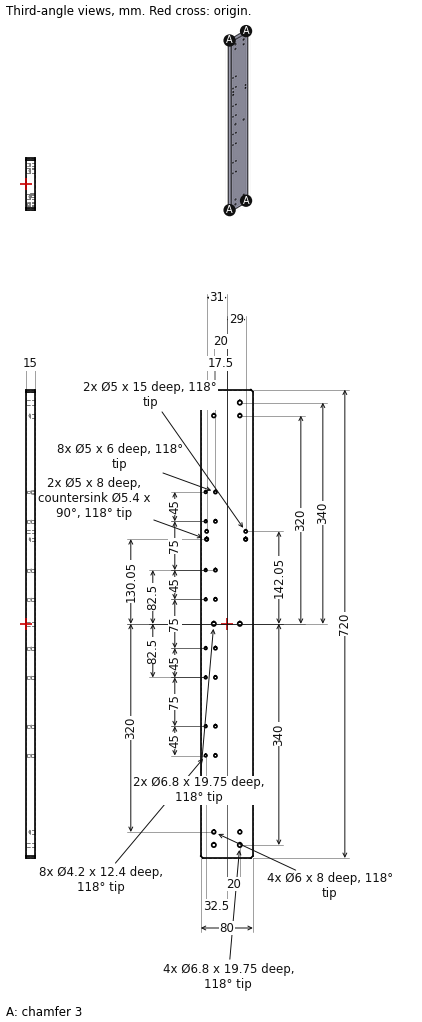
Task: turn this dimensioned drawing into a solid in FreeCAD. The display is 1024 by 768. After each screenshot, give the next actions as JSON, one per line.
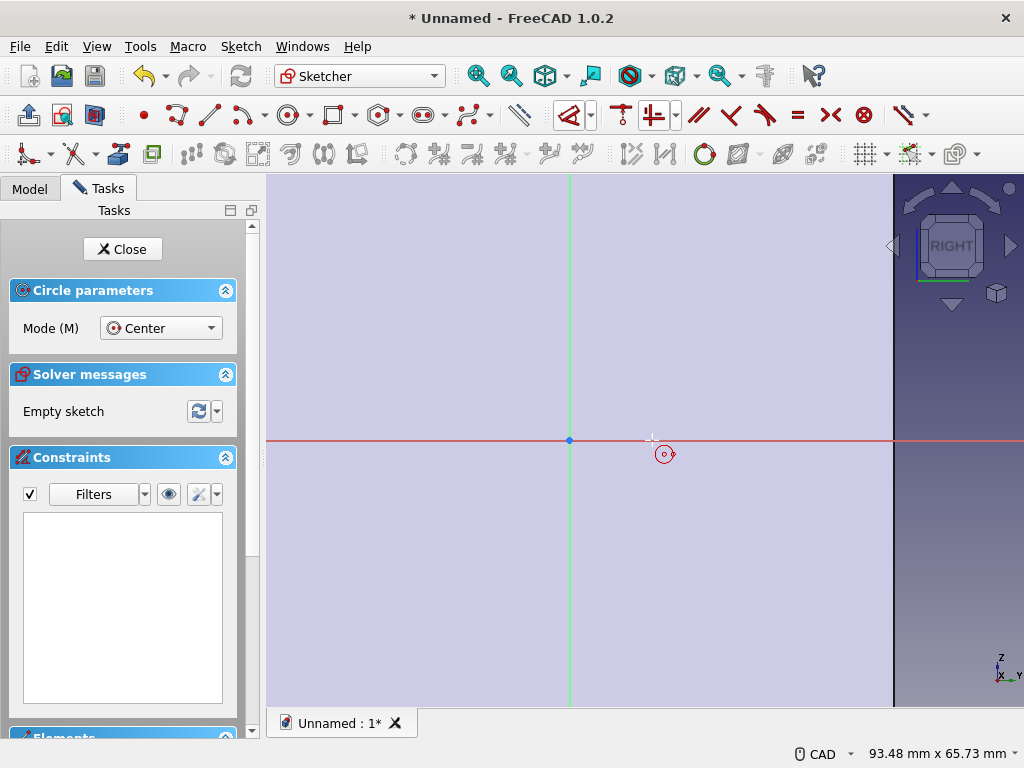
{"action": "left_click", "coordinate": [408, 440]}
{"action": "mouse_move", "coordinate": [427, 421]}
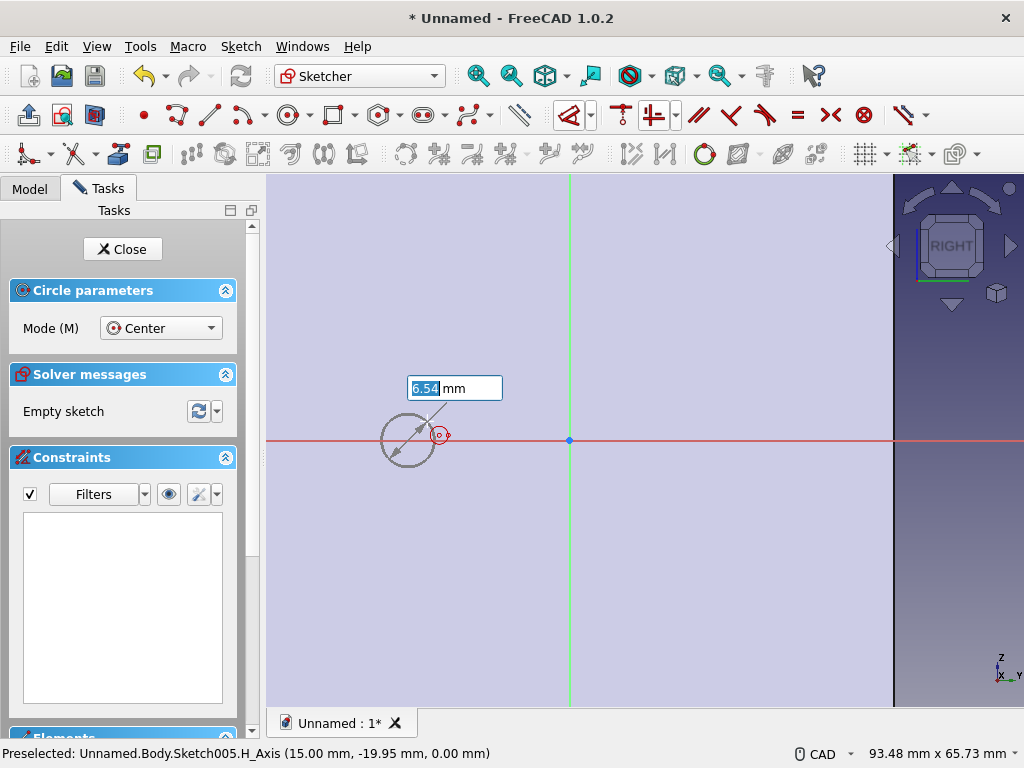
{"action": "type", "text": "6.8"}
{"action": "key", "text": "Return"}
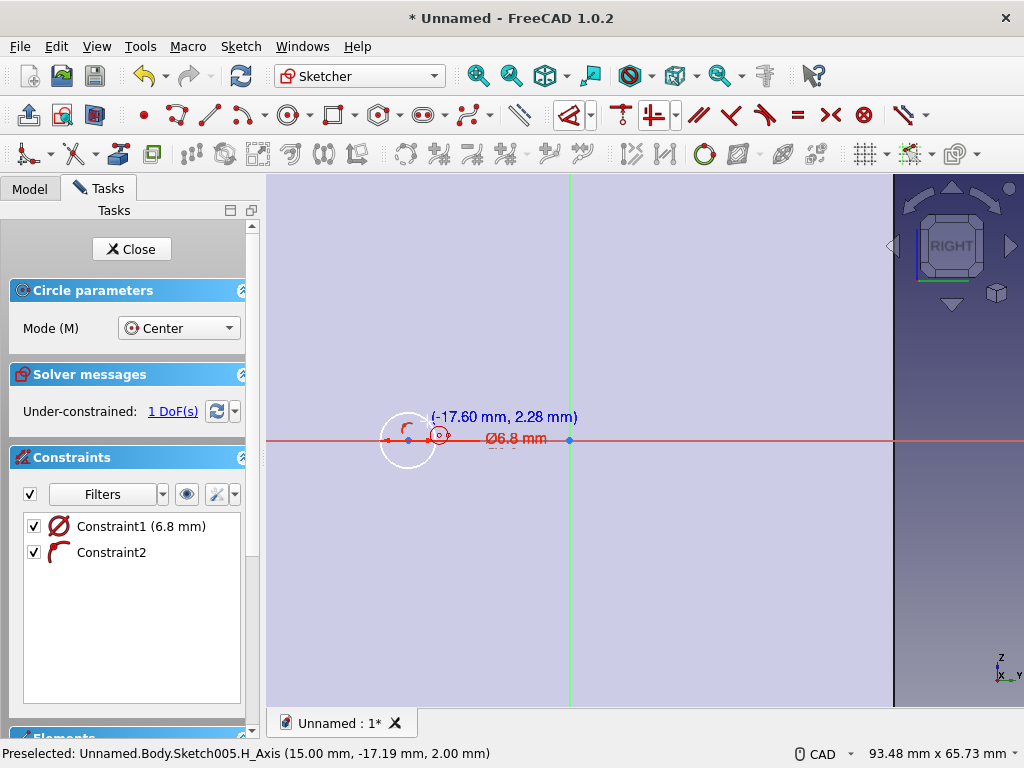
{"action": "left_click", "coordinate": [732, 440]}
{"action": "mouse_move", "coordinate": [751, 421]}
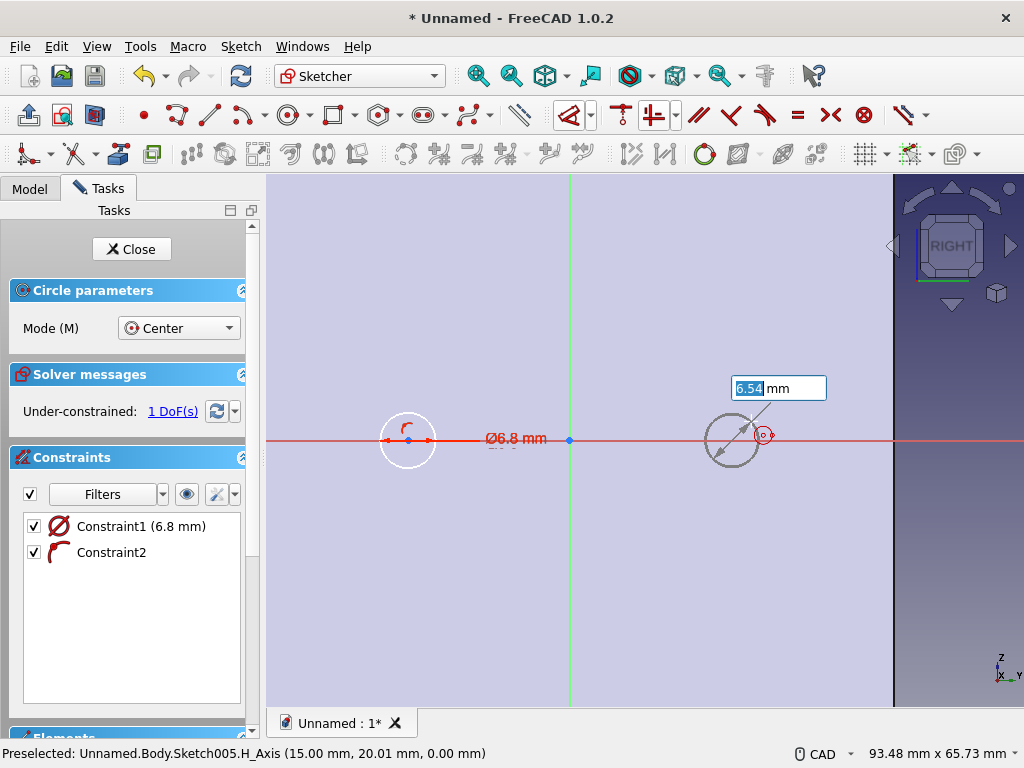
{"action": "type", "text": "6.8"}
{"action": "key", "text": "Return"}
{"action": "key", "text": "Escape"}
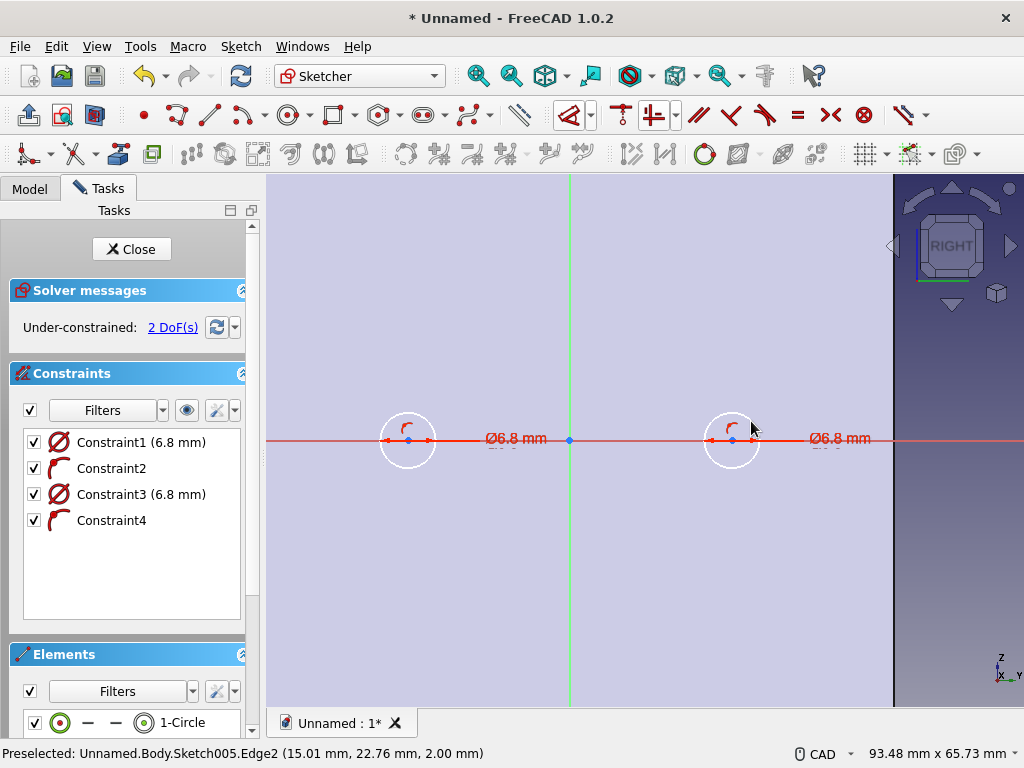
{"action": "left_click", "coordinate": [408, 440]}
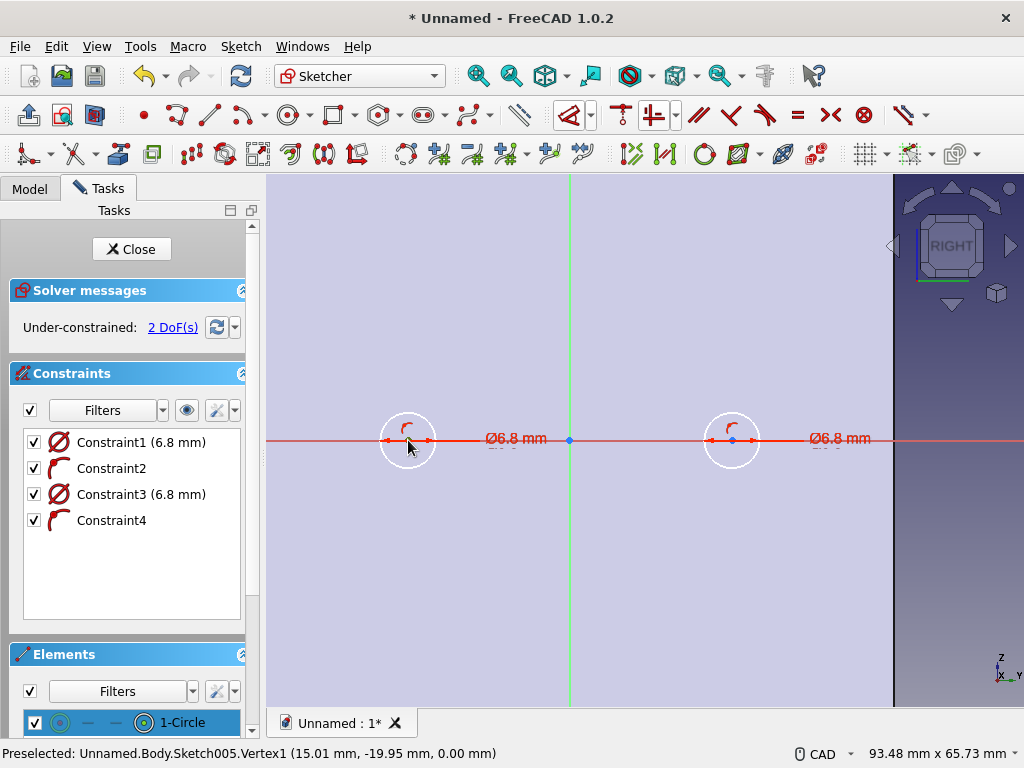
{"action": "left_click", "coordinate": [590, 116]}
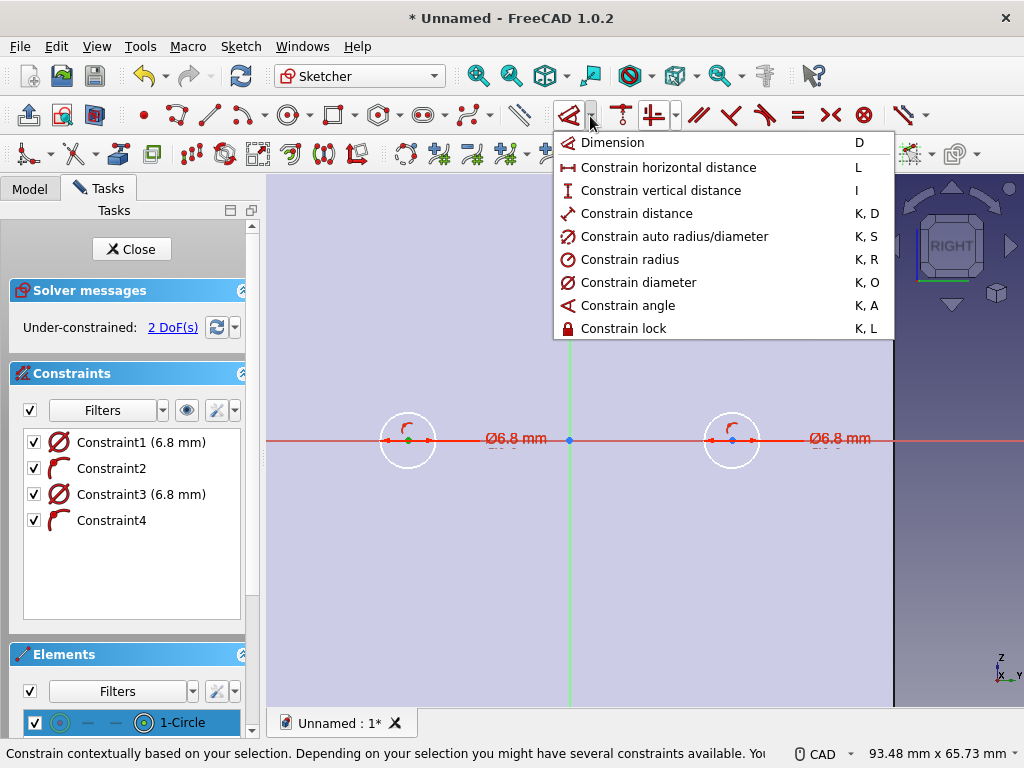
{"action": "left_click", "coordinate": [724, 168]}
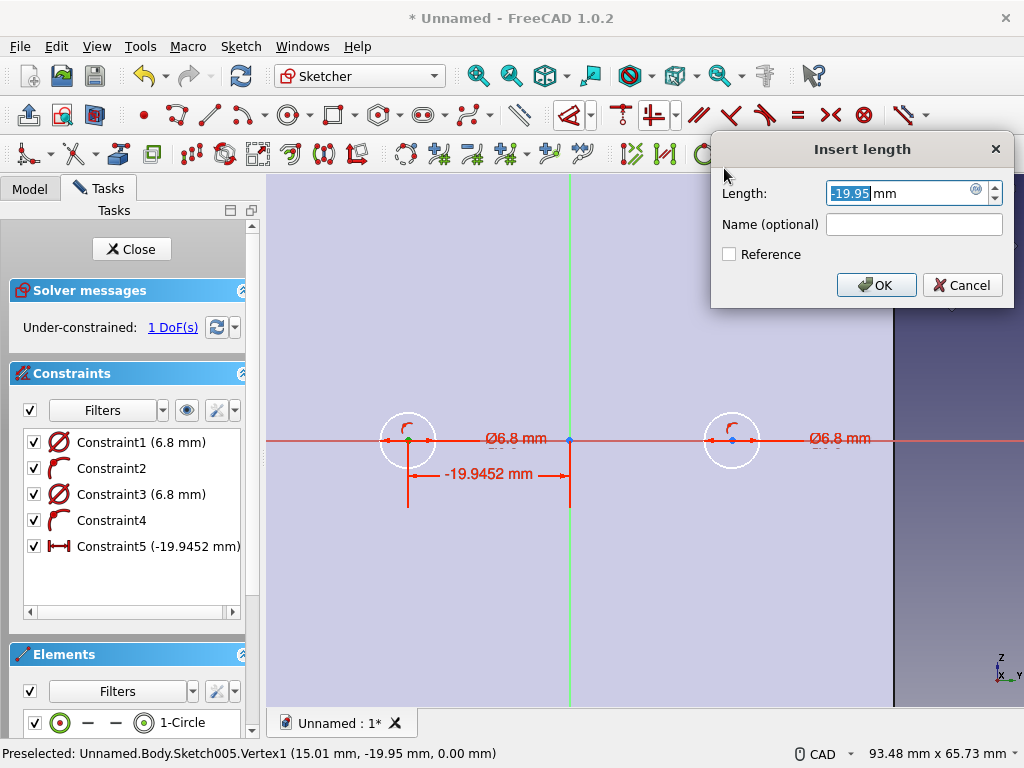
{"action": "type", "text": "-20"}
{"action": "key", "text": "Return"}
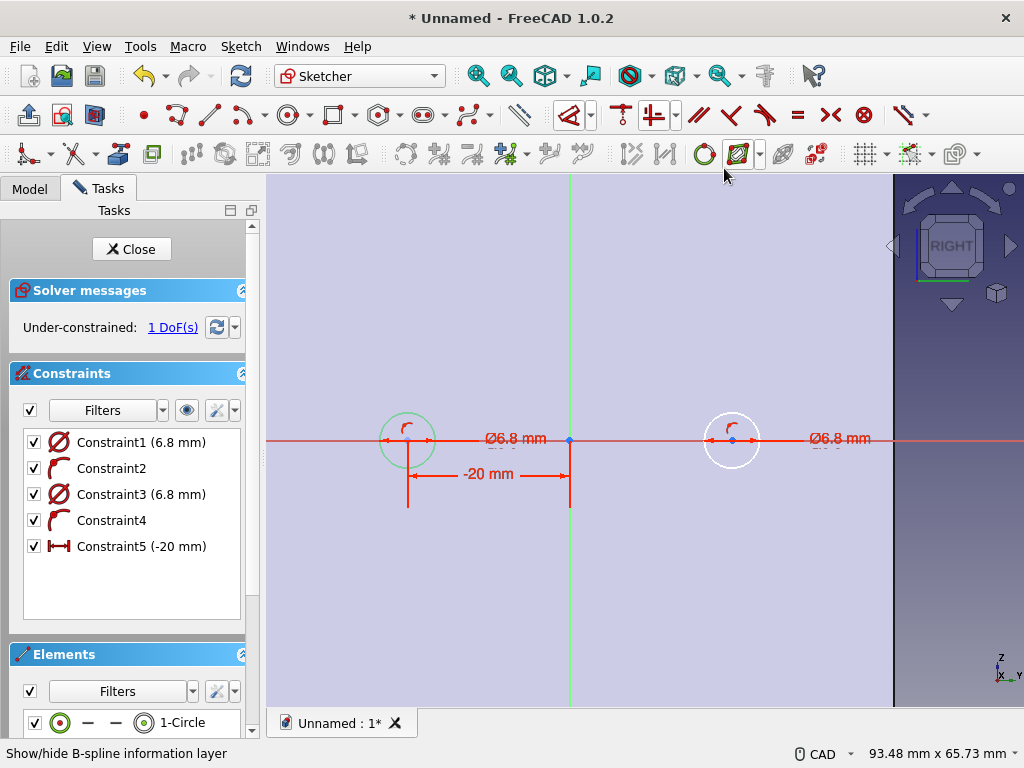
{"action": "left_click", "coordinate": [732, 440]}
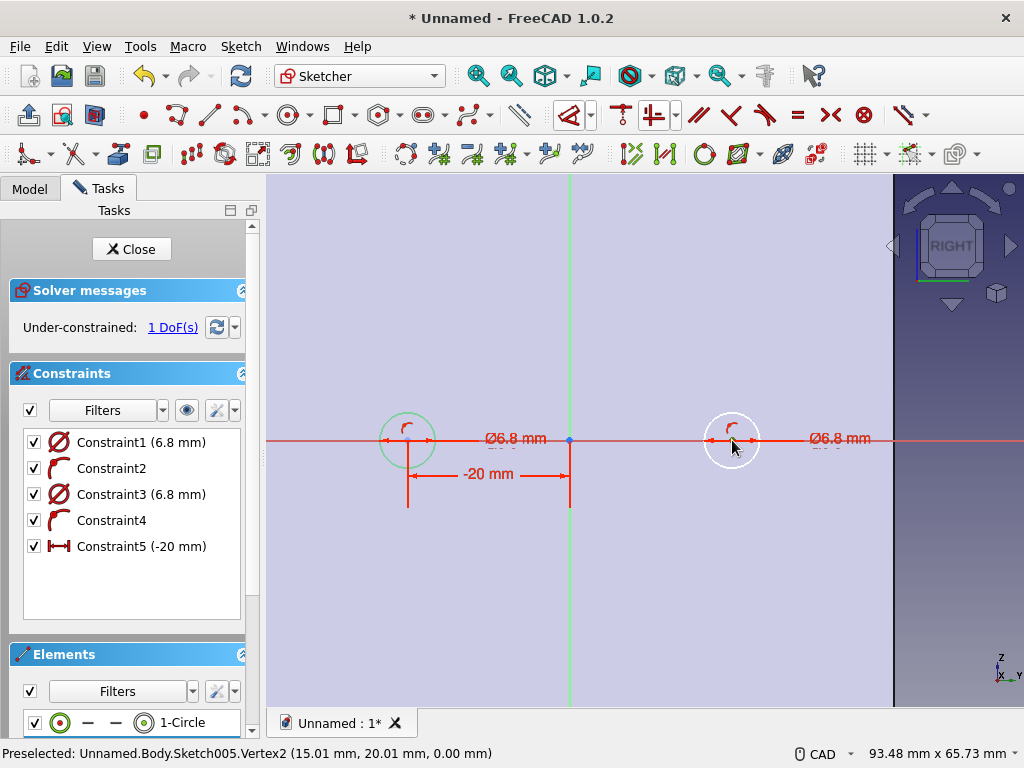
{"action": "key", "text": "l"}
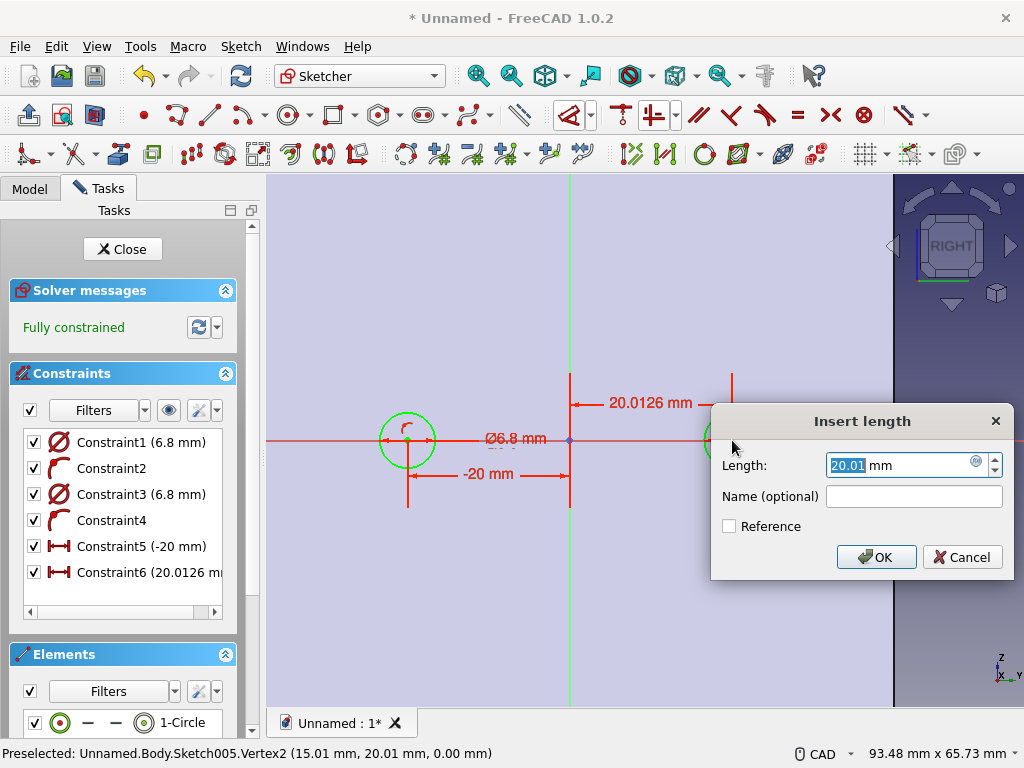
{"action": "type", "text": "20"}
{"action": "key", "text": "Return"}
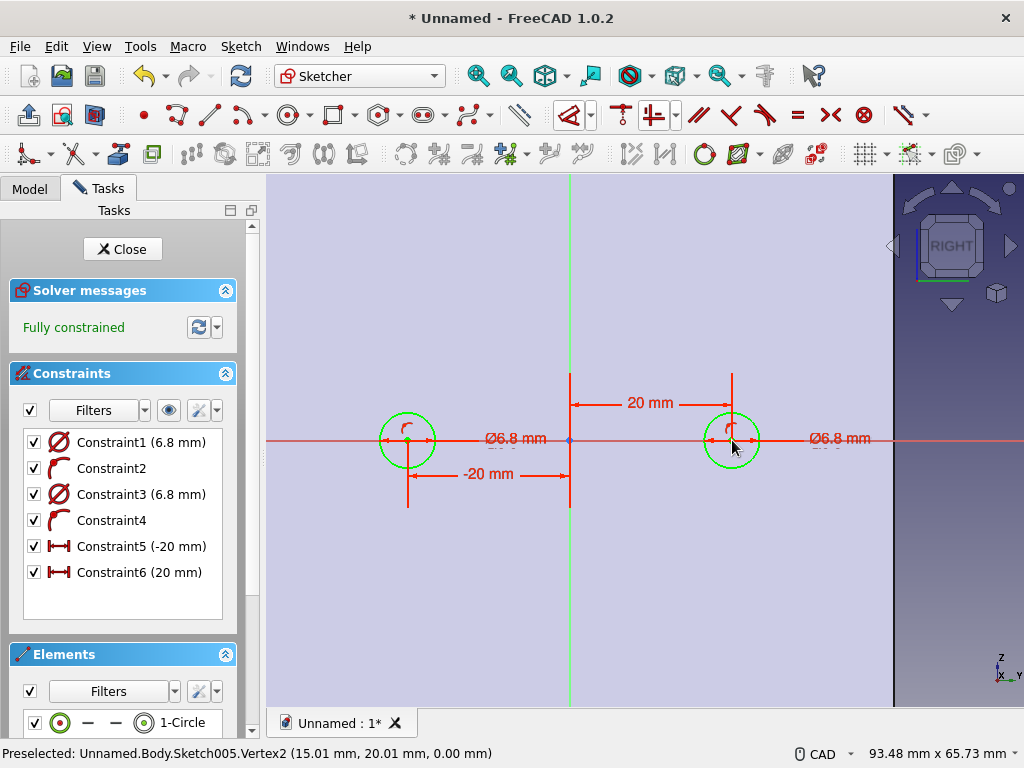
{"action": "left_click", "coordinate": [123, 249]}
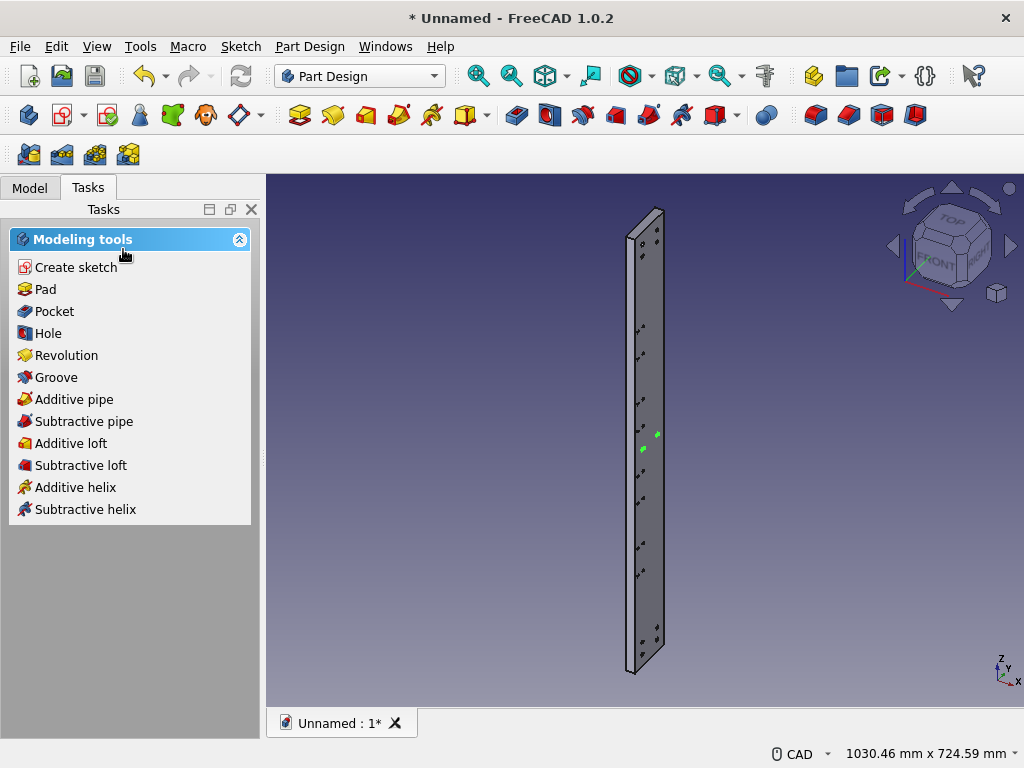
{"action": "left_click", "coordinate": [550, 116]}